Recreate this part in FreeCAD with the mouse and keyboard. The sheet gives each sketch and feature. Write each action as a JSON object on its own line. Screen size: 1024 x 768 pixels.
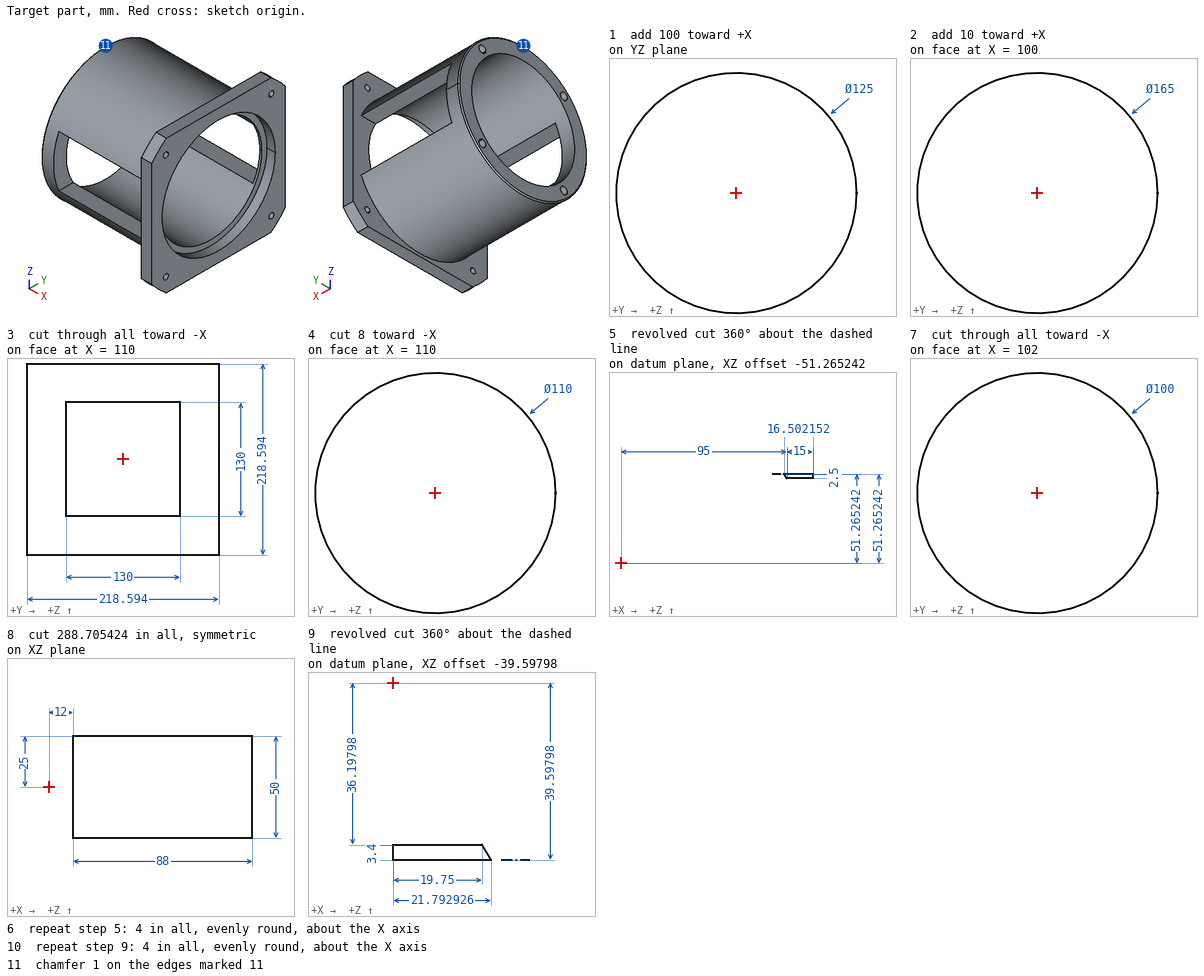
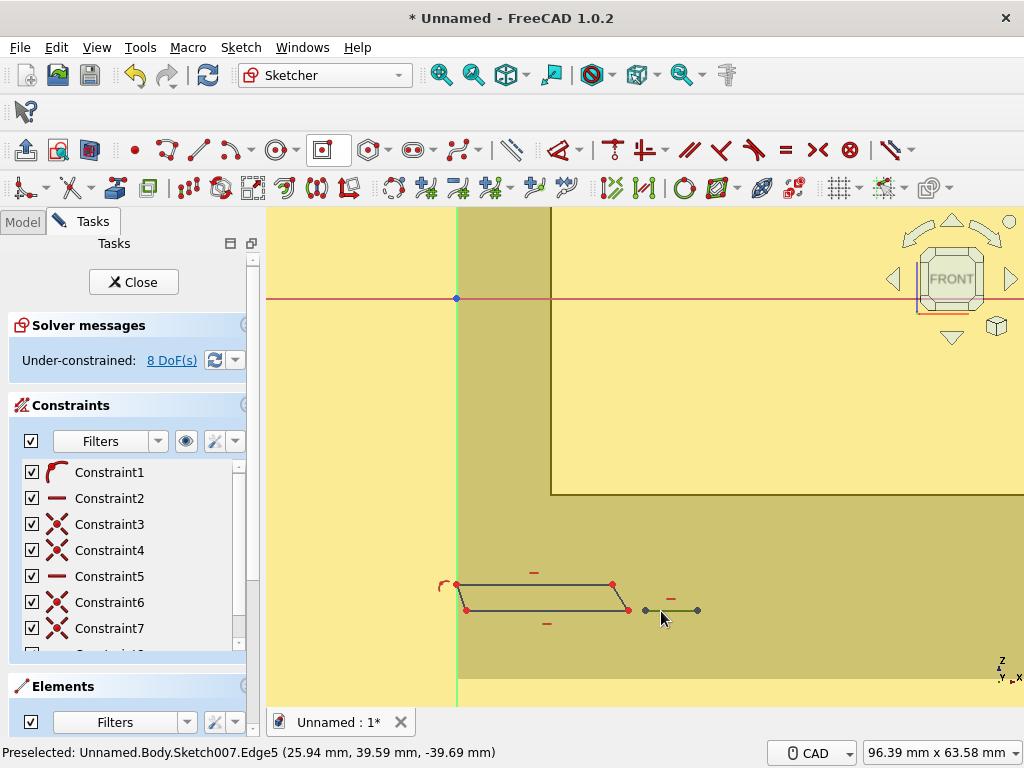
{"action": "left_click", "coordinate": [512, 150]}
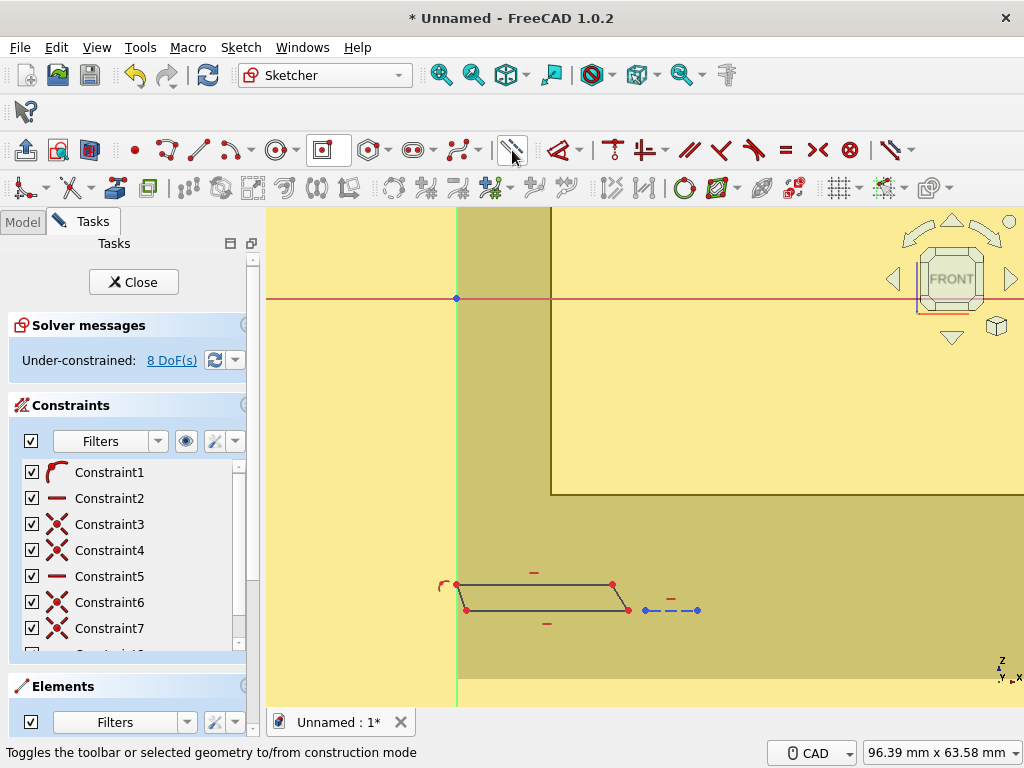
{"action": "scroll", "coordinate": [461, 595], "scroll_direction": "up", "scroll_amount": 2}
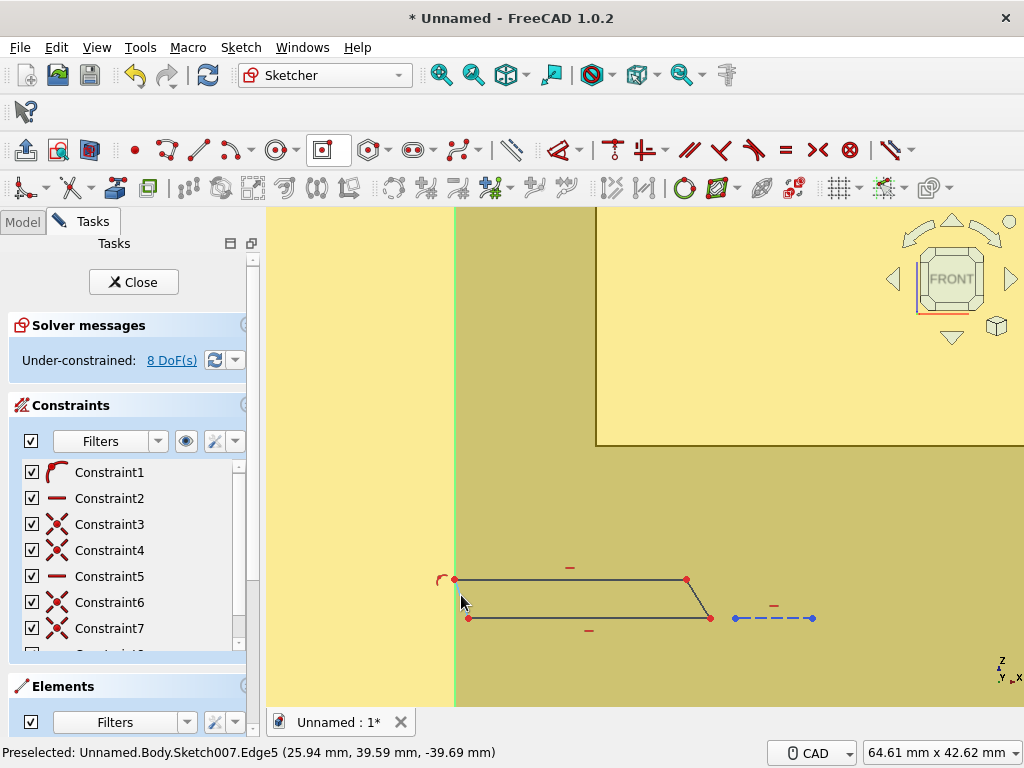
{"action": "left_click", "coordinate": [460, 595]}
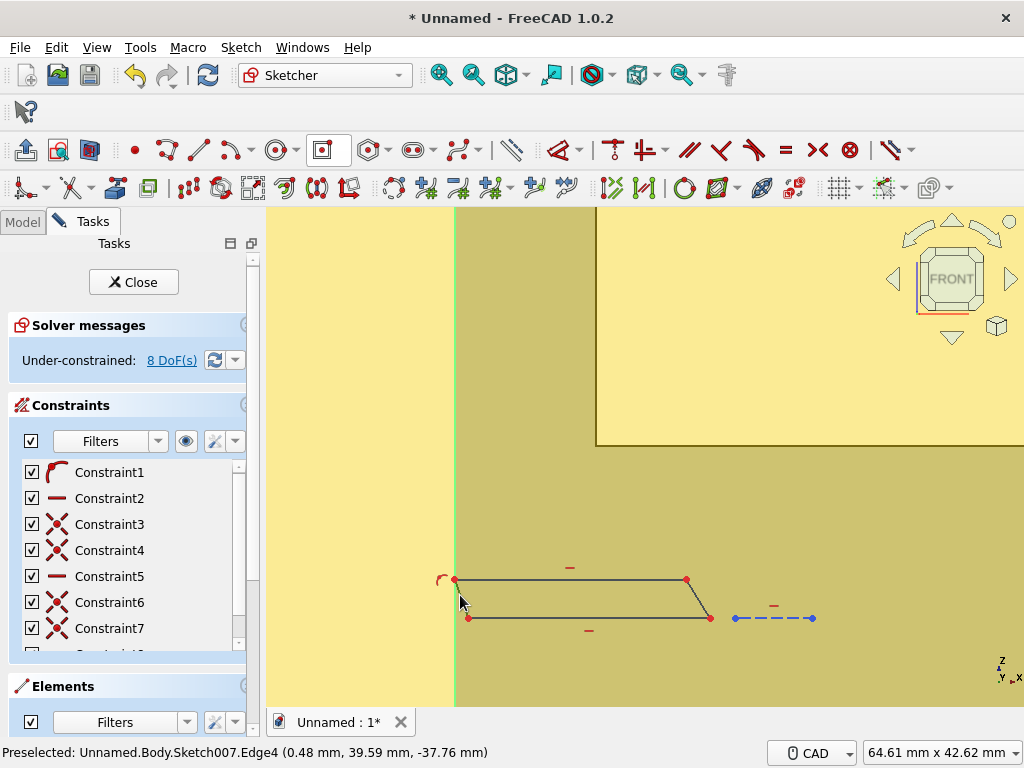
{"action": "left_click", "coordinate": [668, 150]}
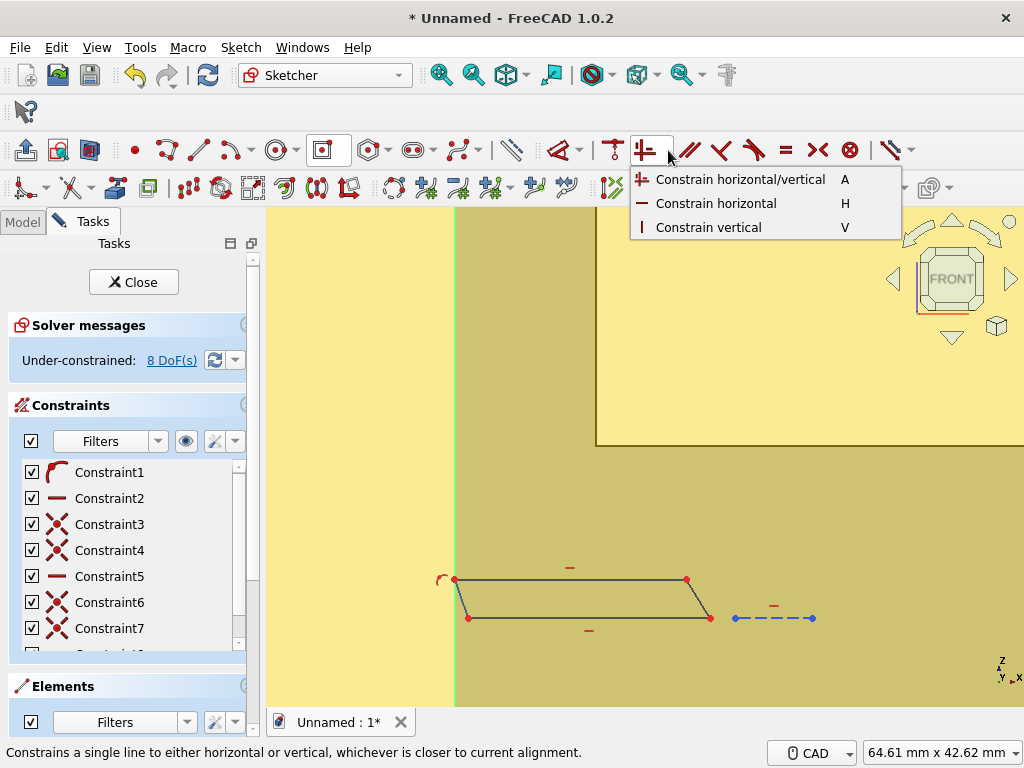
{"action": "left_click", "coordinate": [766, 227]}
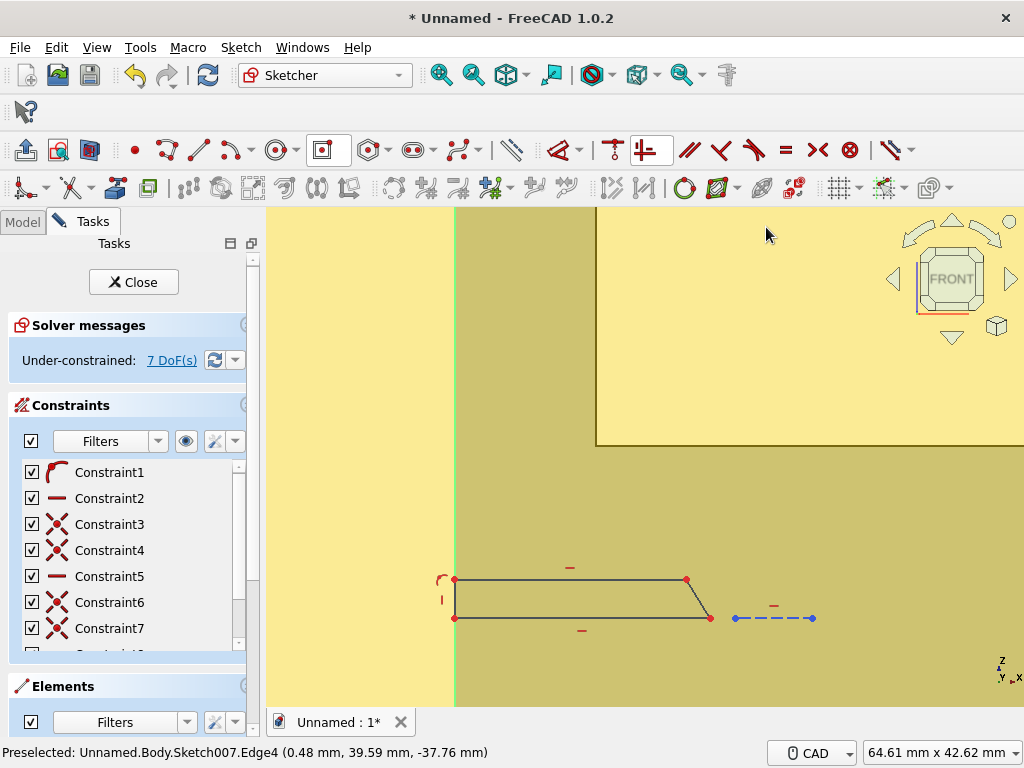
{"action": "left_click", "coordinate": [558, 150]}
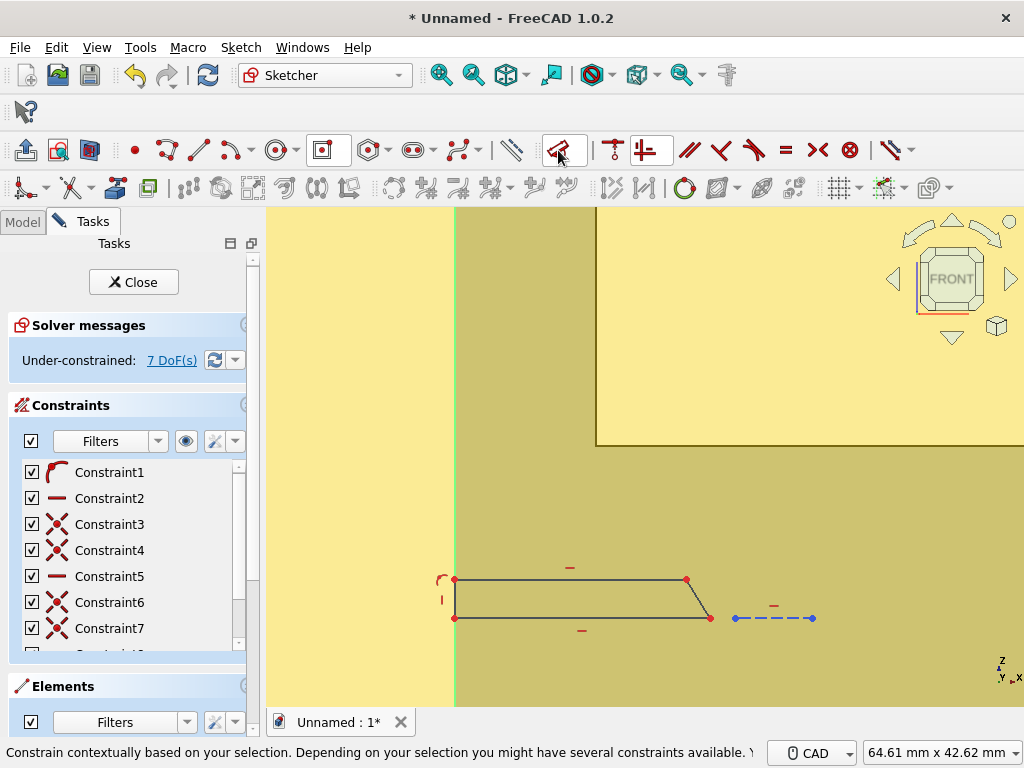
{"action": "left_click", "coordinate": [455, 607]}
{"action": "left_click", "coordinate": [421, 599]}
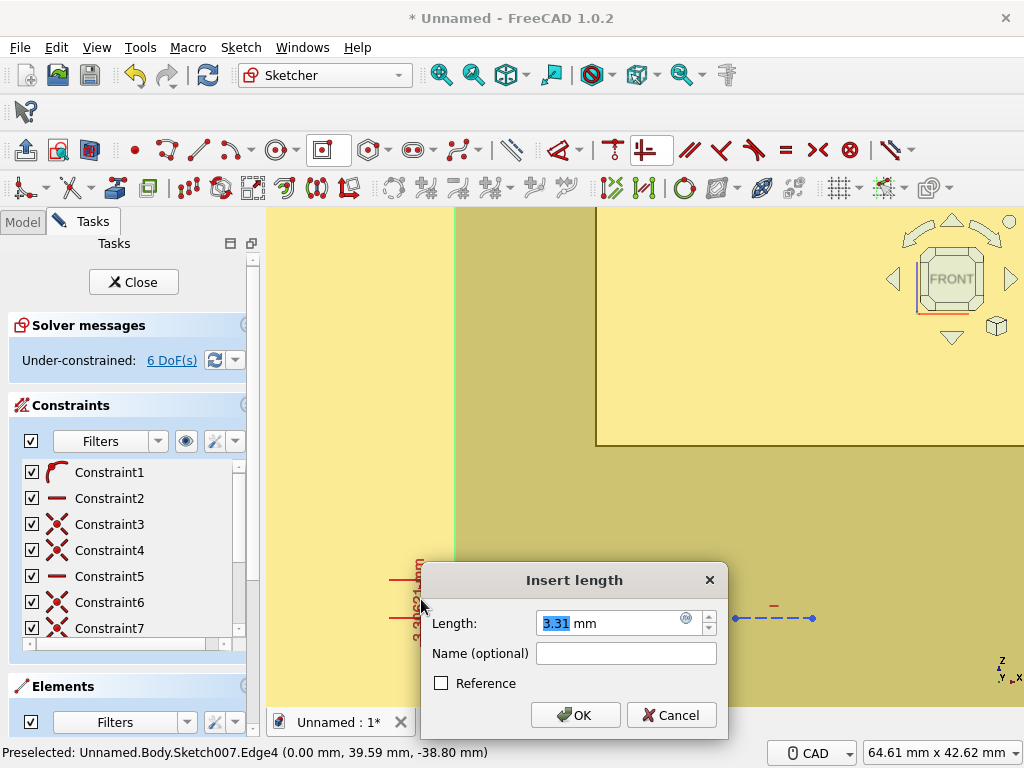
{"action": "type", "text": "3.4"}
{"action": "key", "text": "Return"}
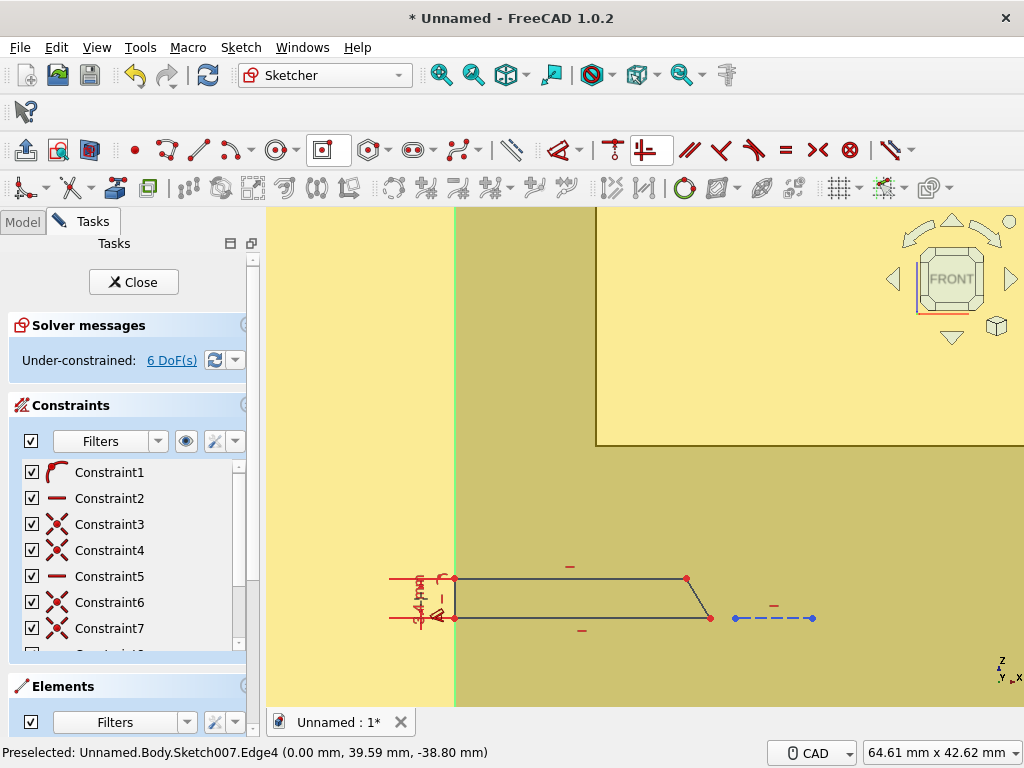
{"action": "left_click", "coordinate": [524, 579]}
{"action": "left_click", "coordinate": [571, 545]}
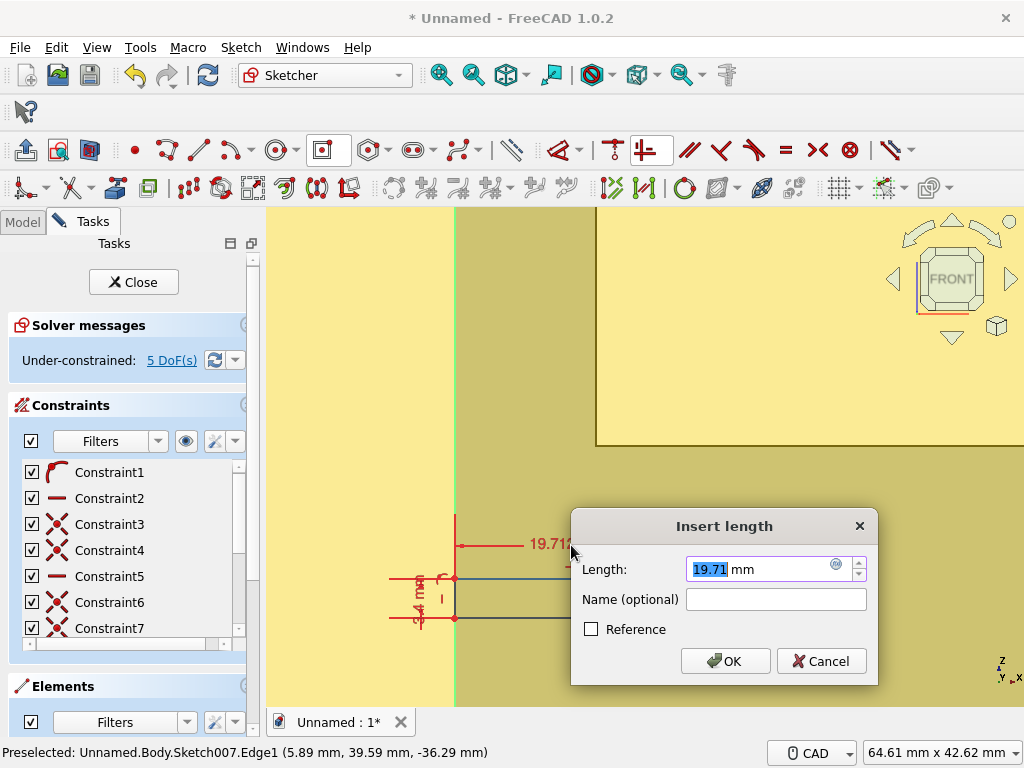
{"action": "type", "text": "19.75"}
{"action": "key", "text": "Return"}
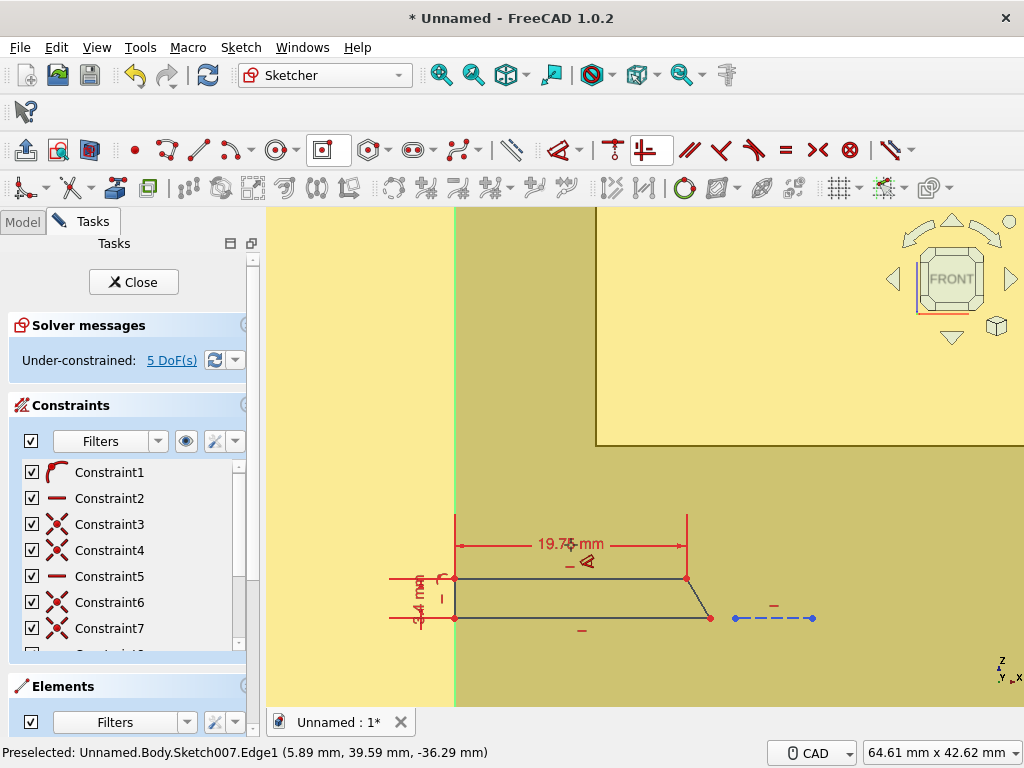
{"action": "left_click", "coordinate": [633, 618]}
{"action": "left_click", "coordinate": [582, 652]}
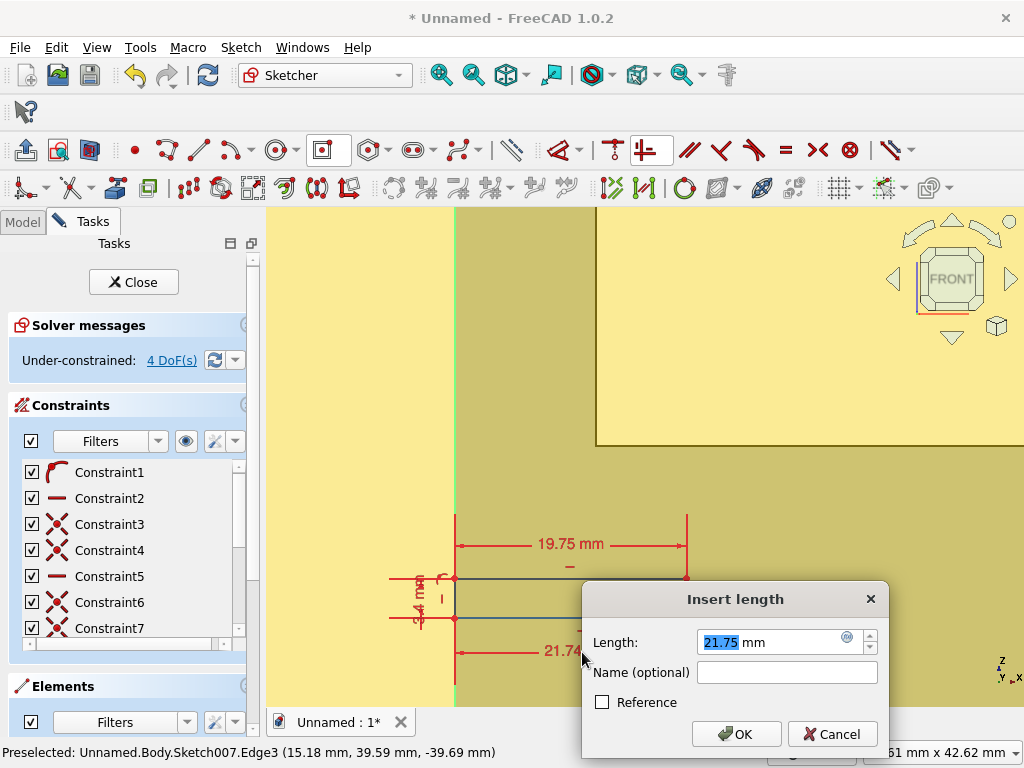
{"action": "type", "text": "21.792926"}
{"action": "key", "text": "Return"}